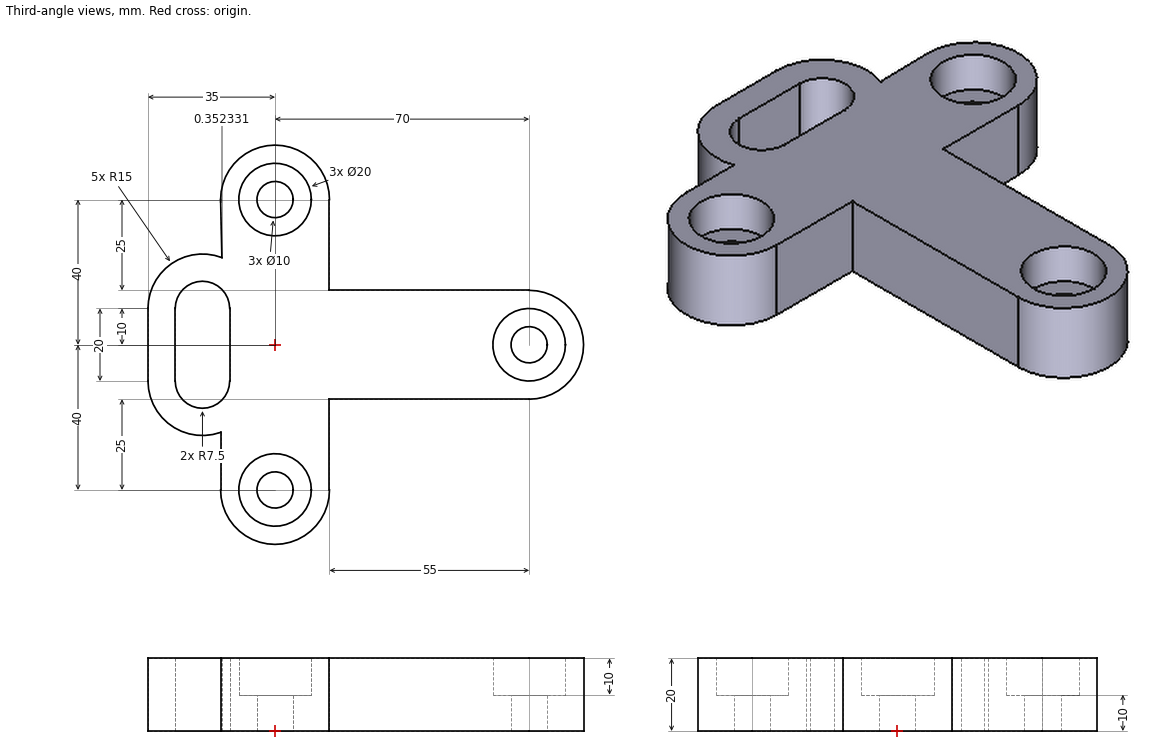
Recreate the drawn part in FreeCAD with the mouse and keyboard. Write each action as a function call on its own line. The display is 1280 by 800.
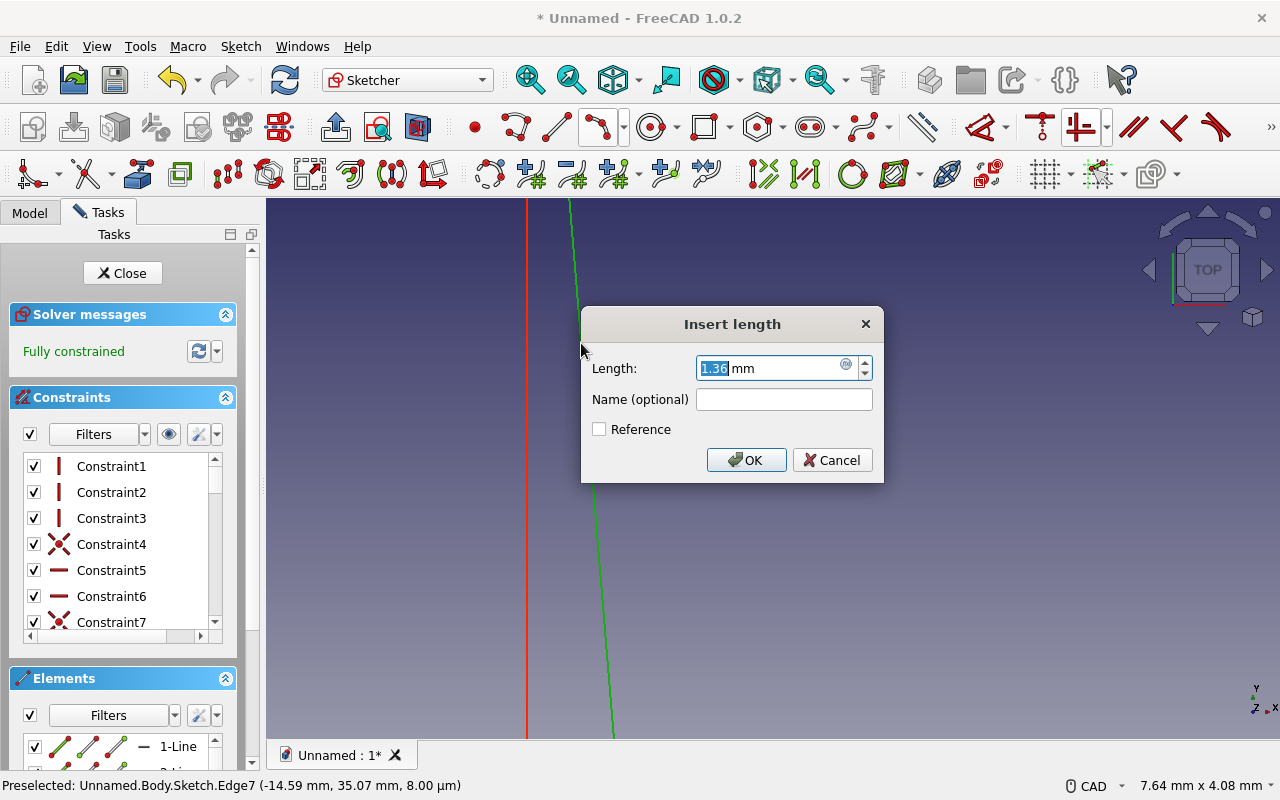
text(0.352331)
key(Return)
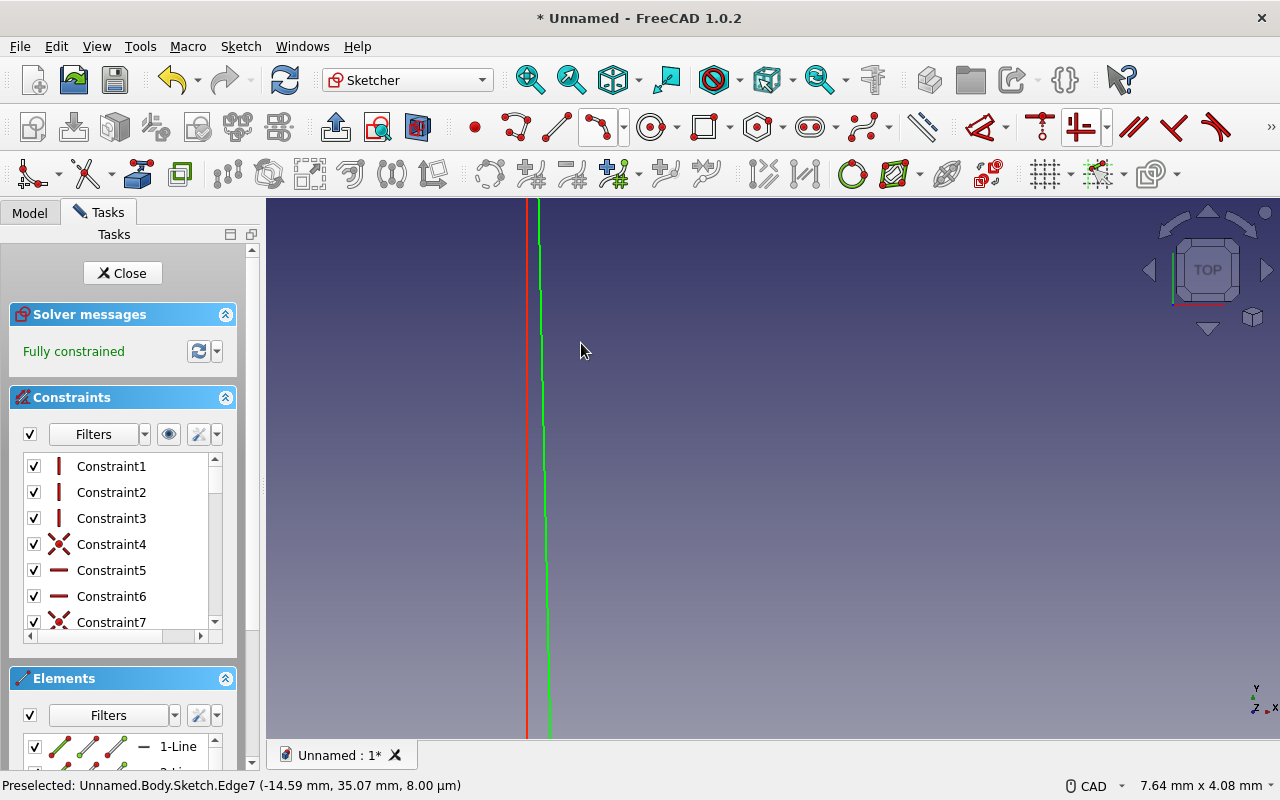
click(123, 273)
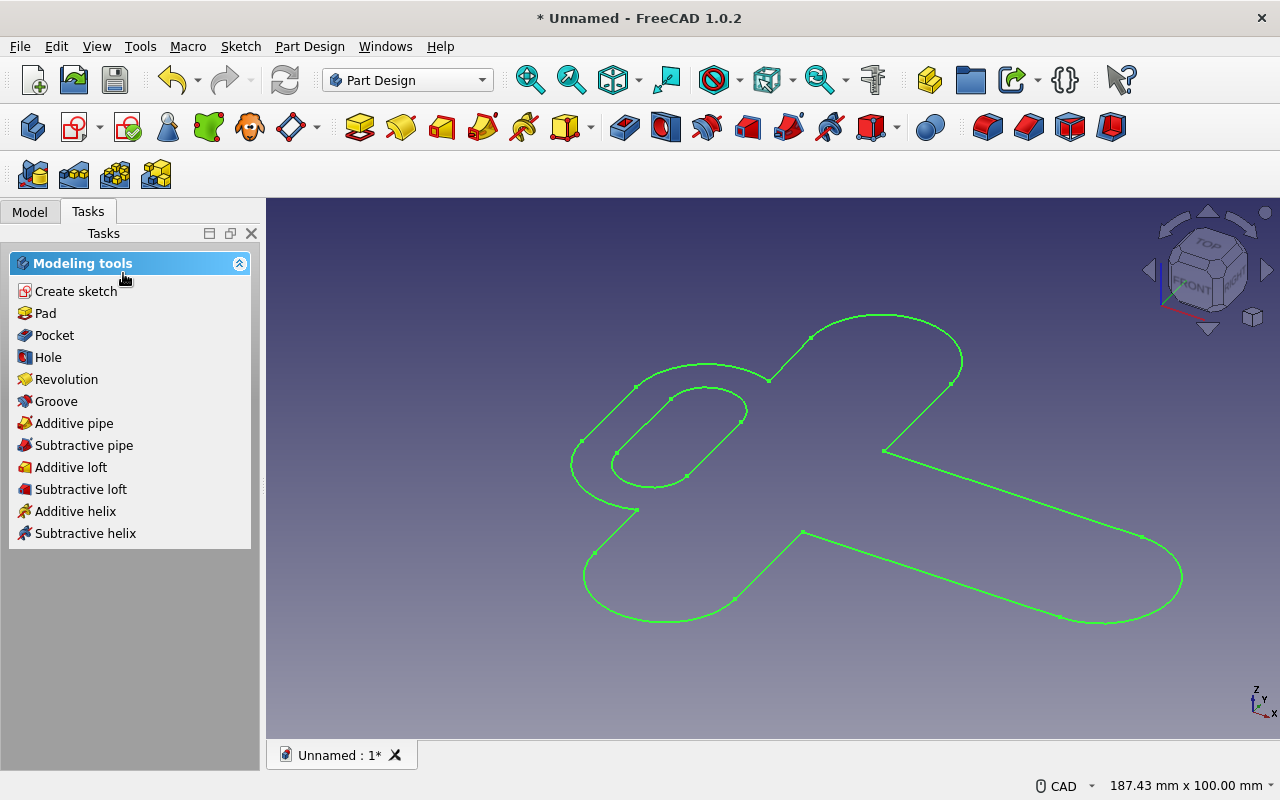
click(360, 128)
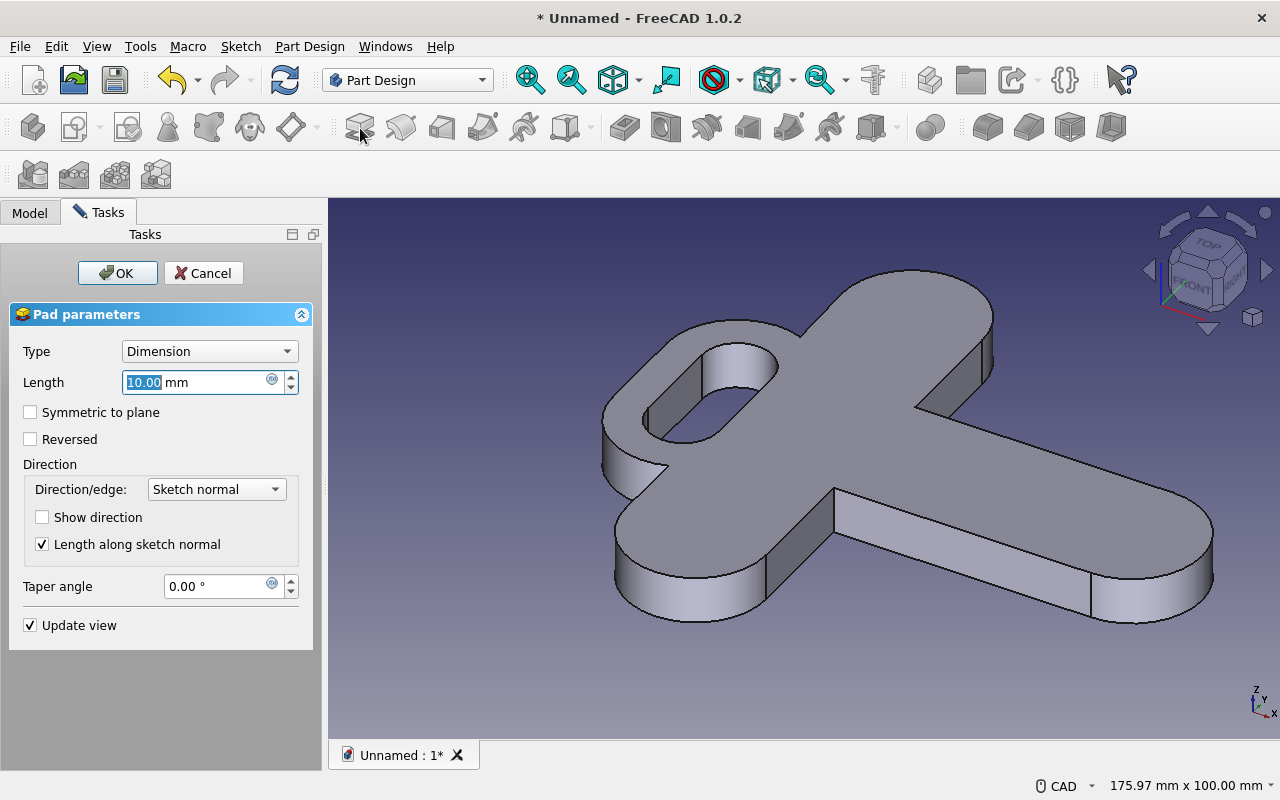
text(20)
key(Tab)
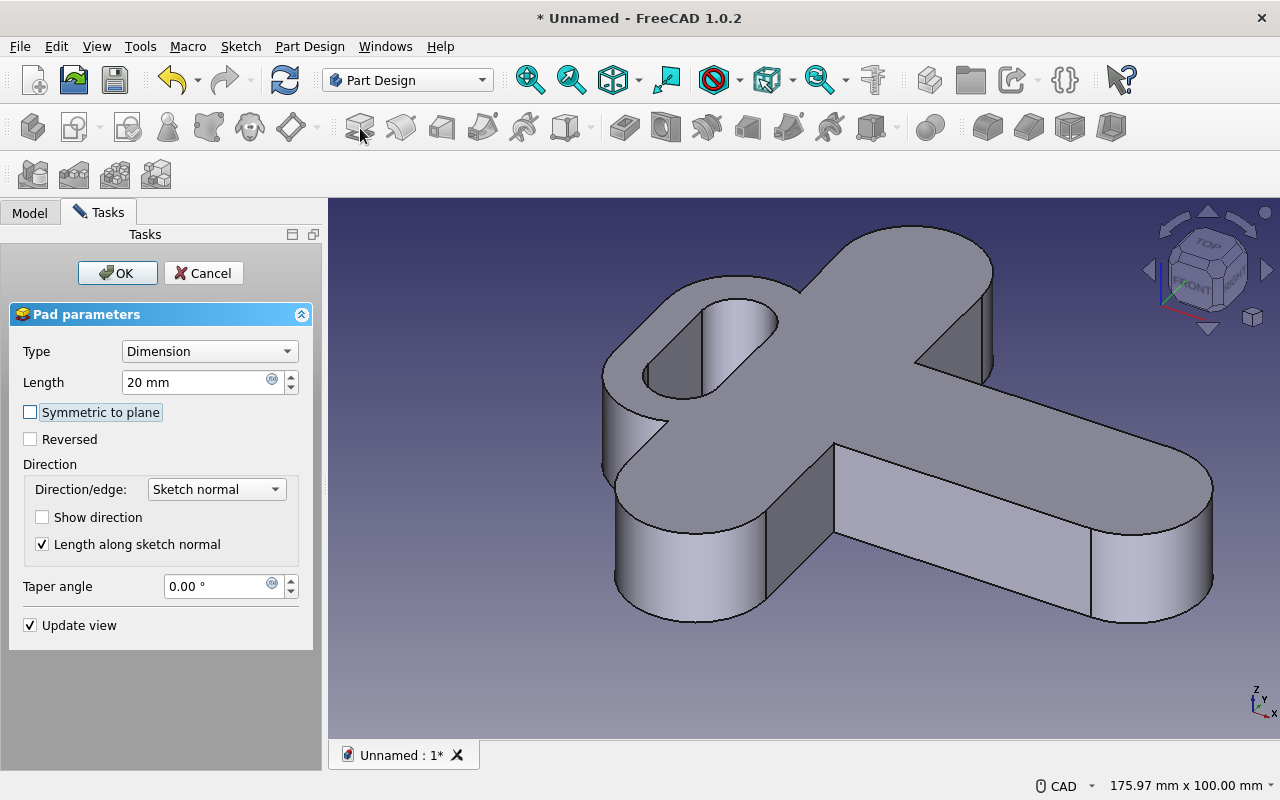
click(118, 273)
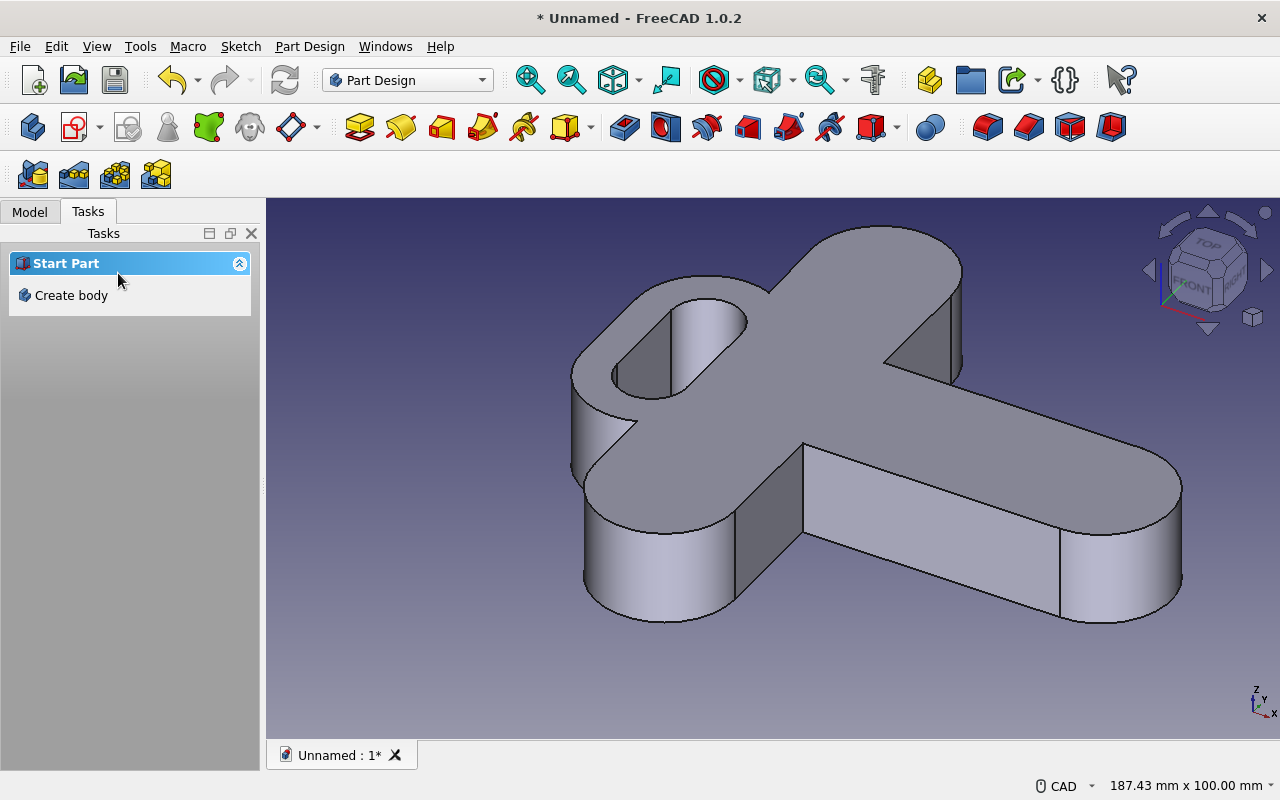
click(531, 80)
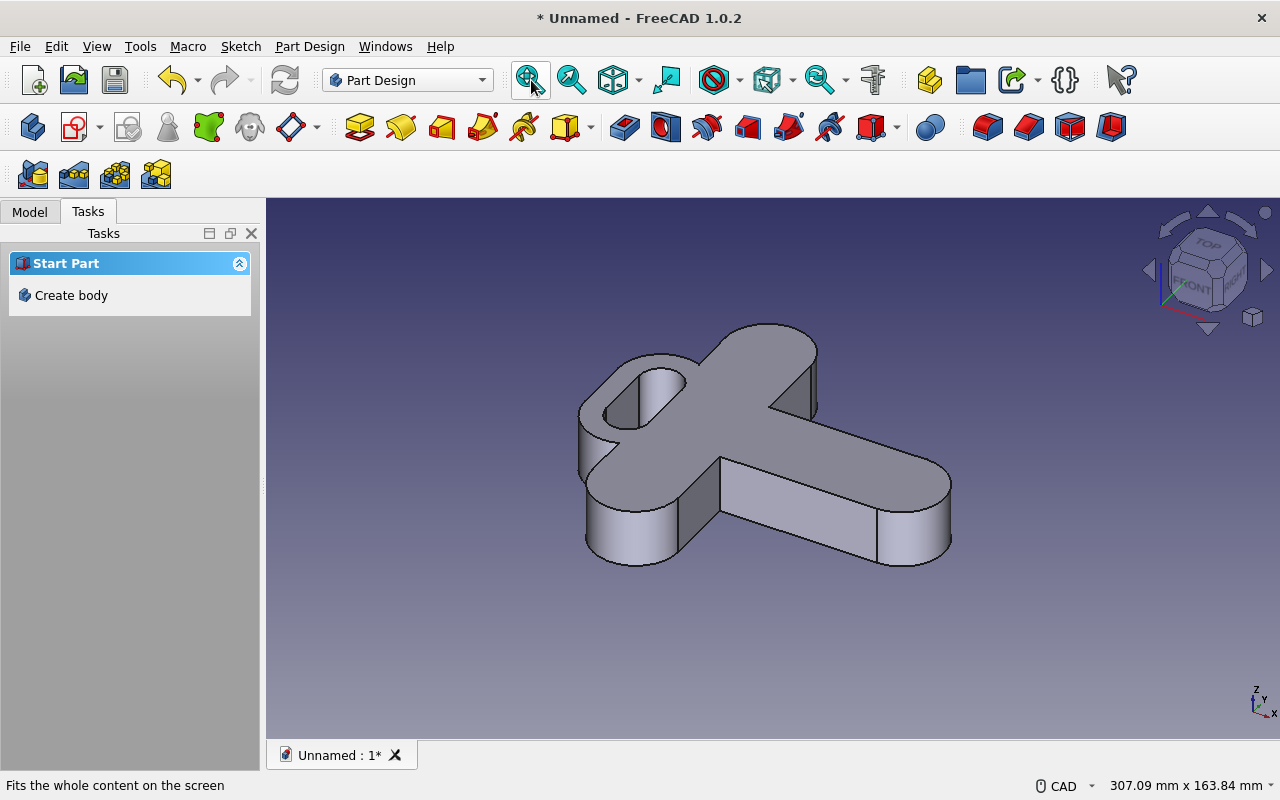
click(724, 424)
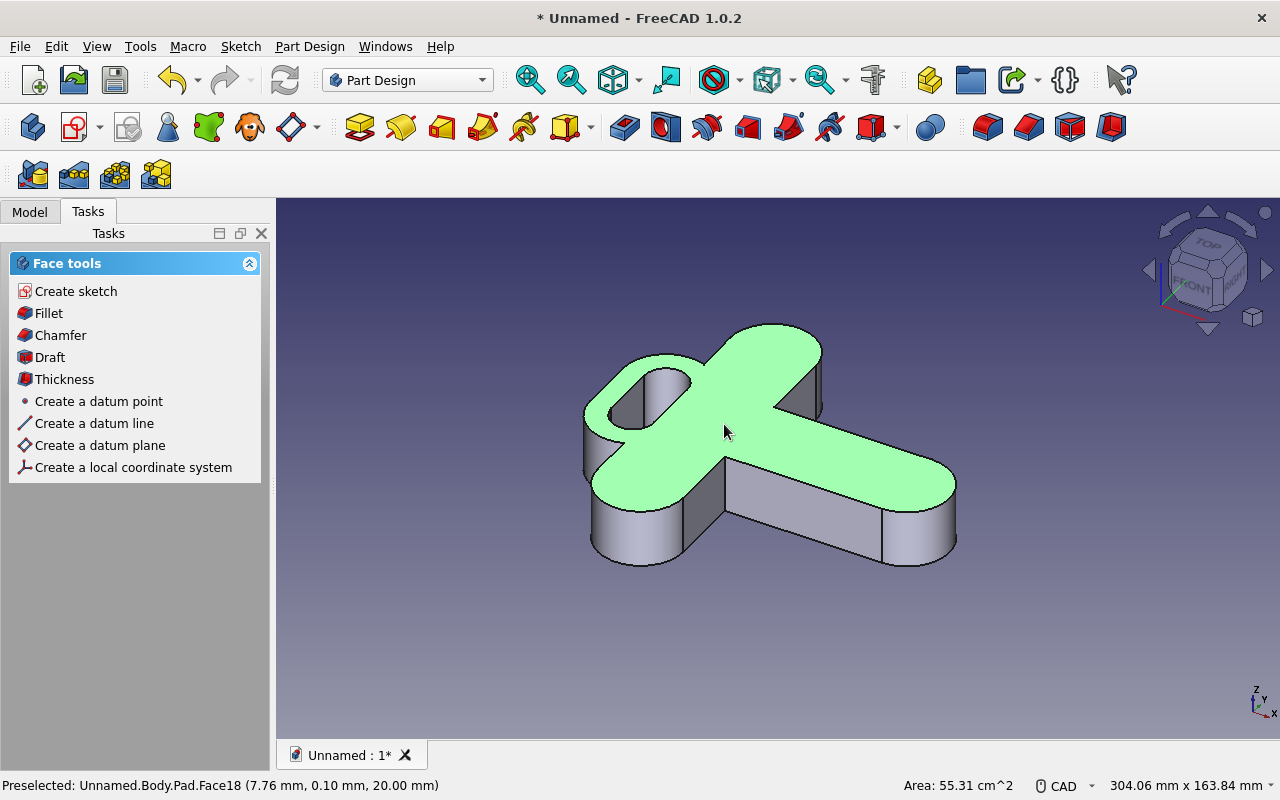
click(74, 128)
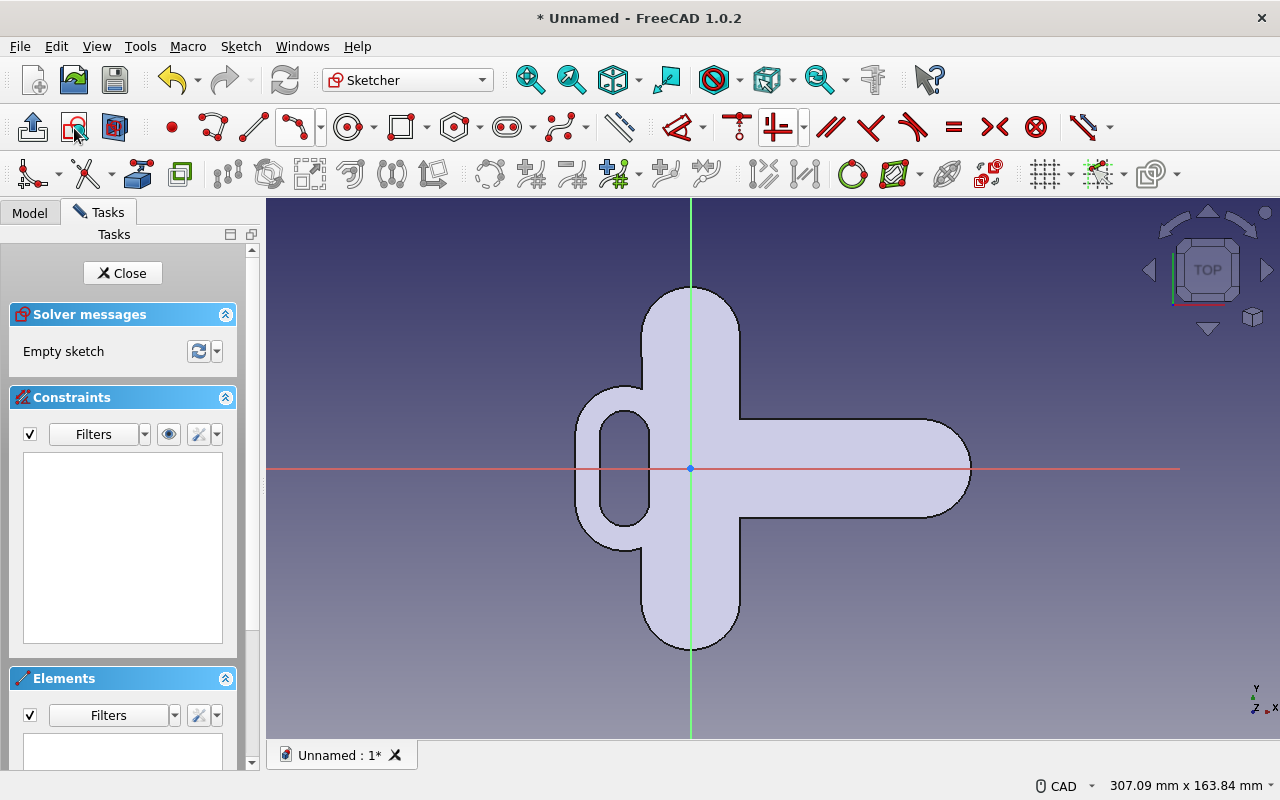
click(348, 128)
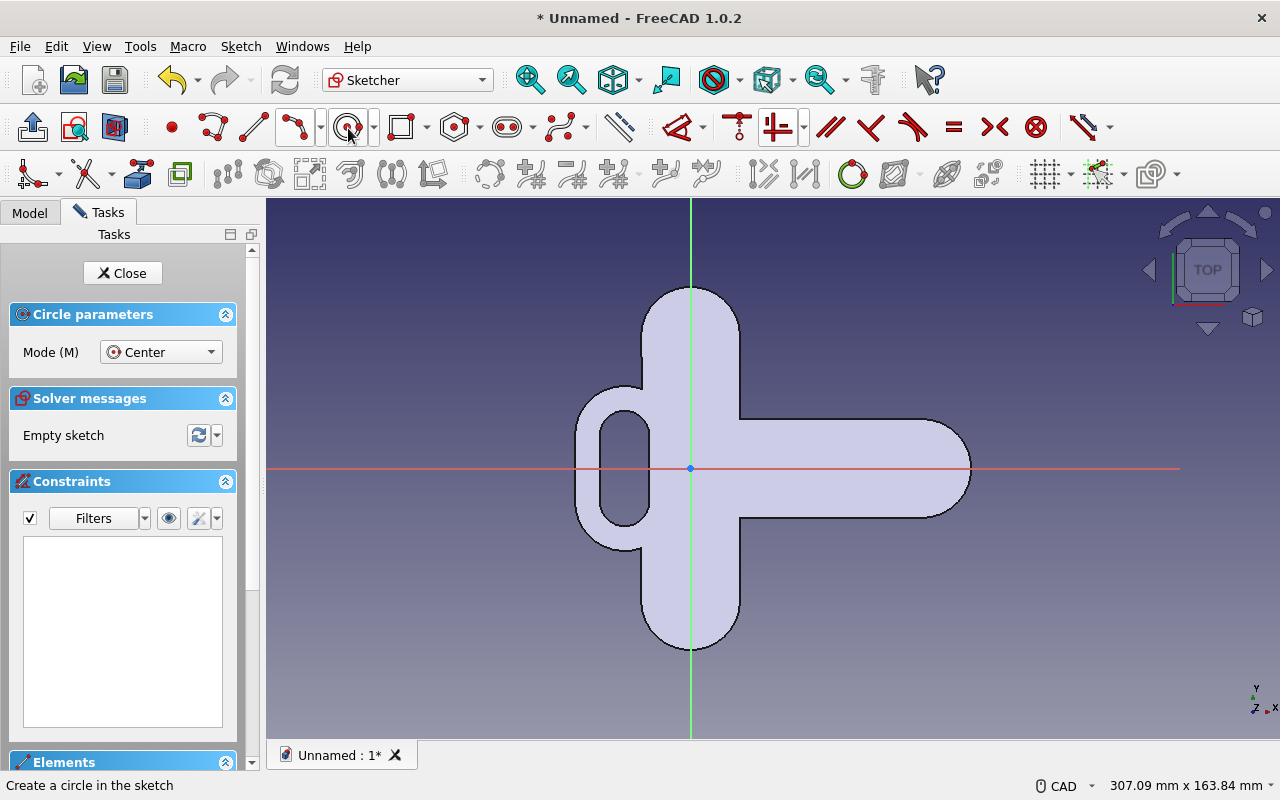
click(691, 336)
move(714, 313)